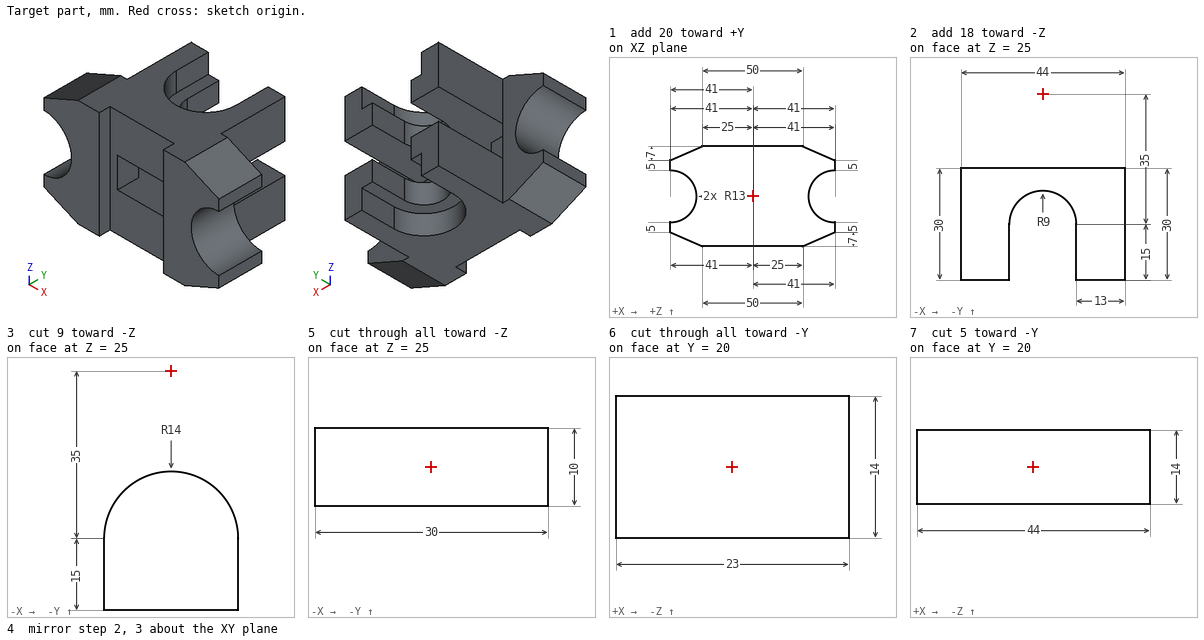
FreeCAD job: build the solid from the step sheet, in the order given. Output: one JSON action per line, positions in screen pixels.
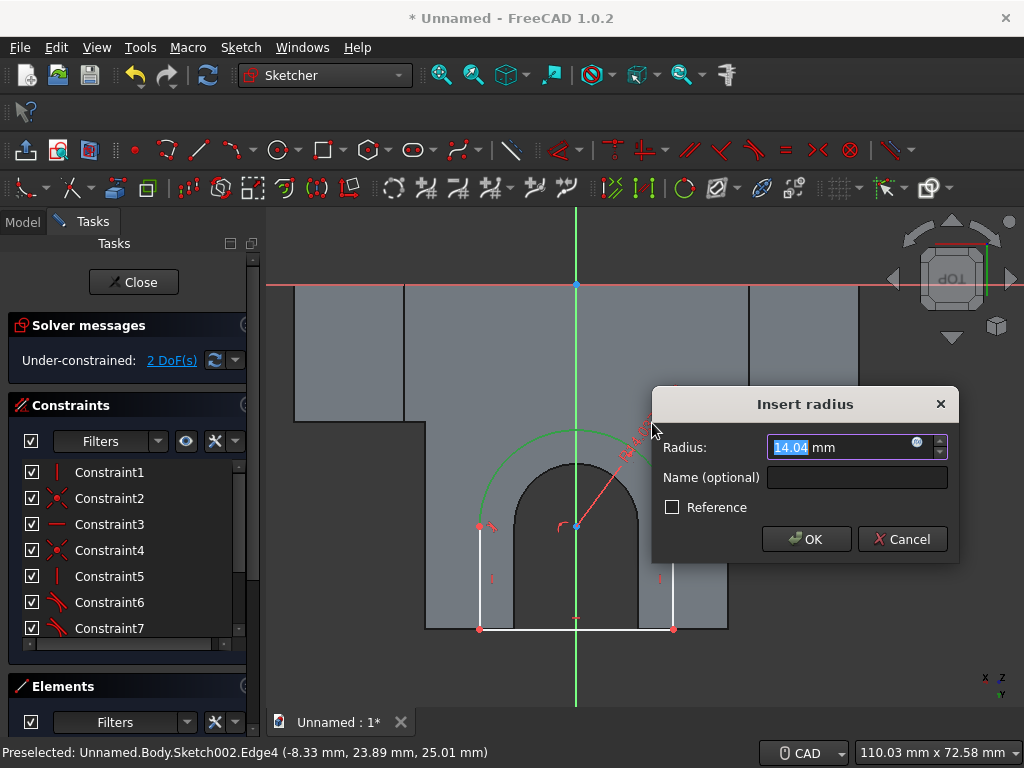
{"action": "type", "text": "14"}
{"action": "key", "text": "Return"}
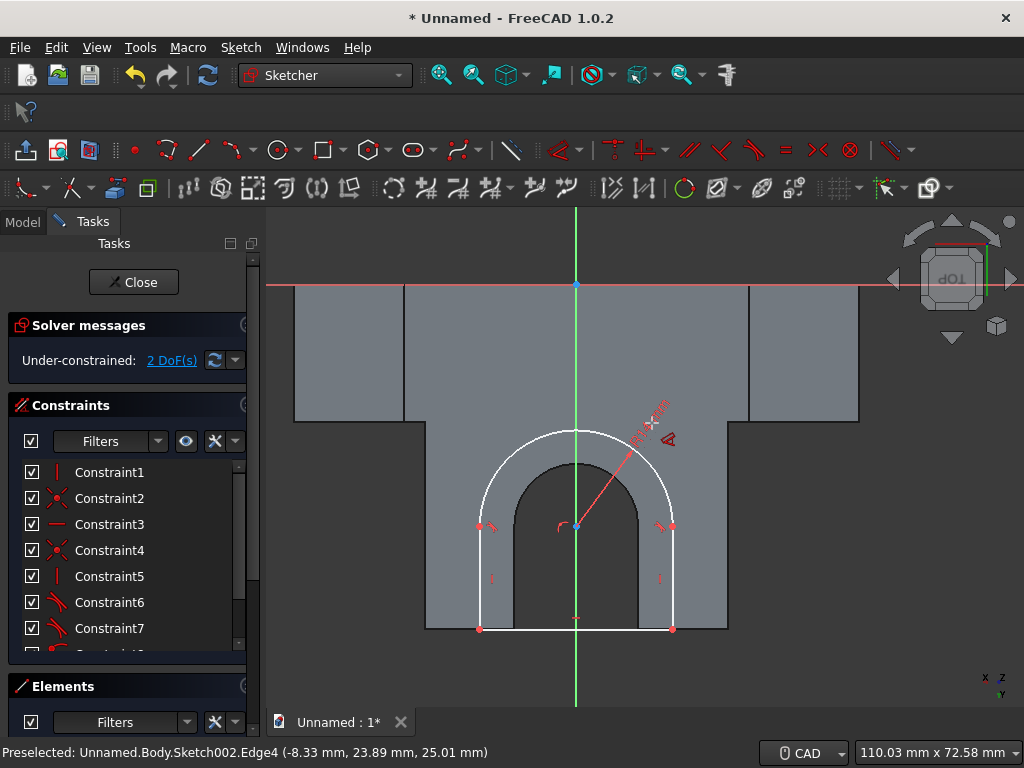
{"action": "left_click", "coordinate": [480, 558]}
{"action": "left_click", "coordinate": [446, 578]}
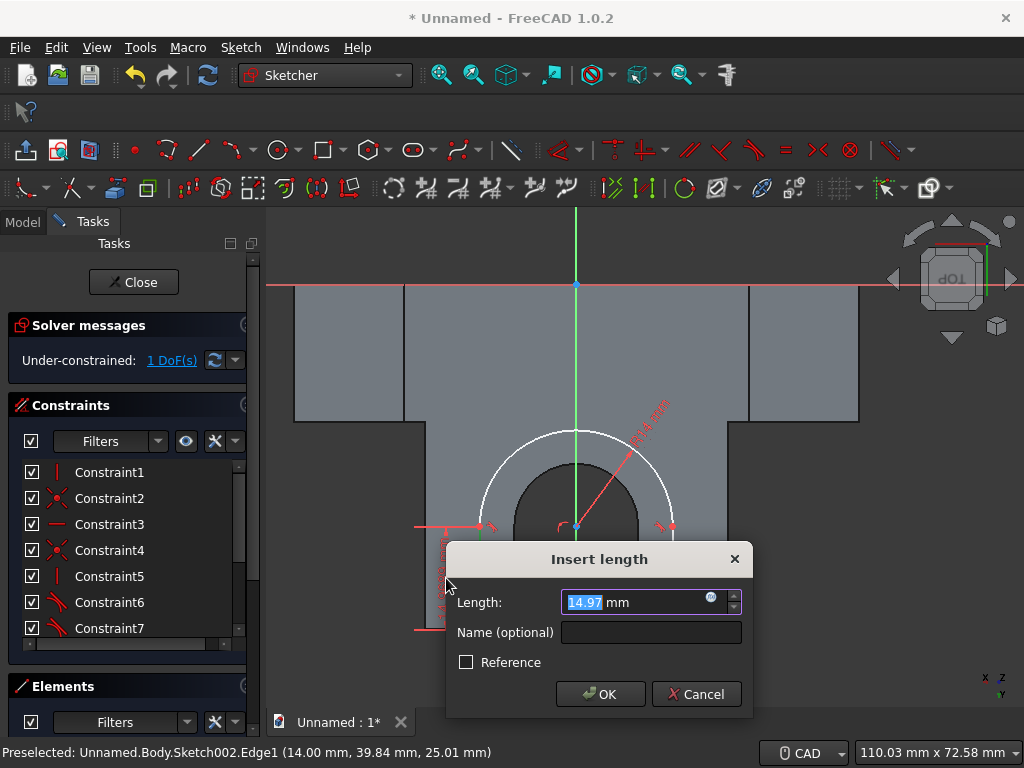
{"action": "type", "text": "15"}
{"action": "key", "text": "Return"}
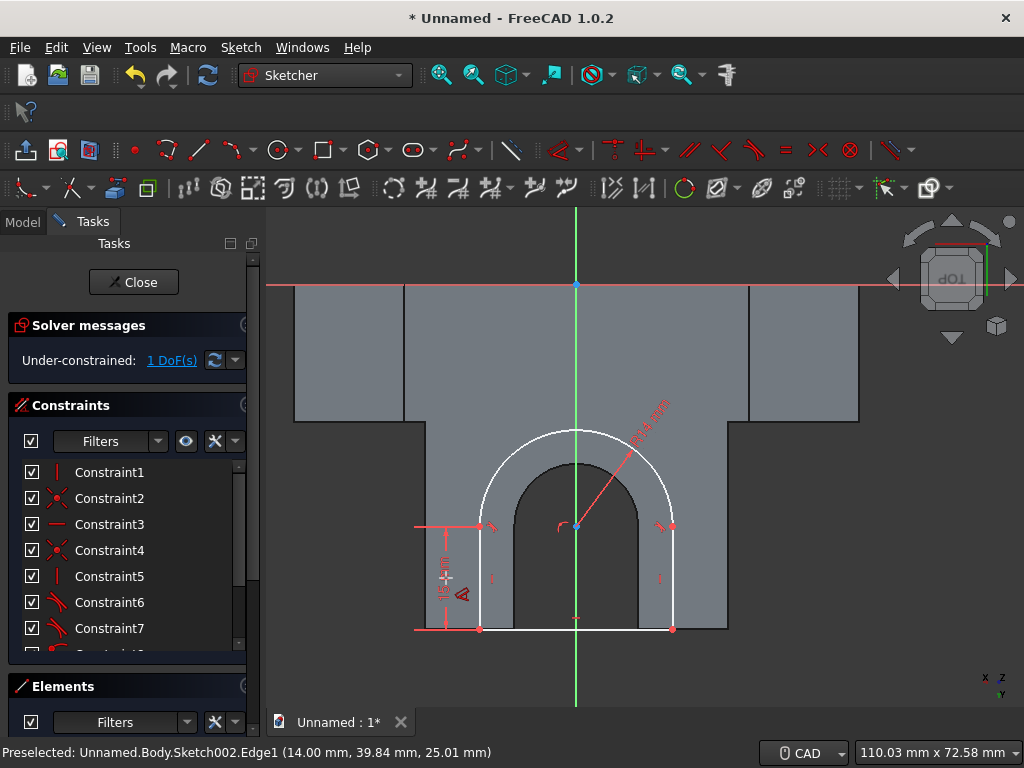
{"action": "left_click", "coordinate": [480, 527]}
{"action": "left_click", "coordinate": [446, 406]}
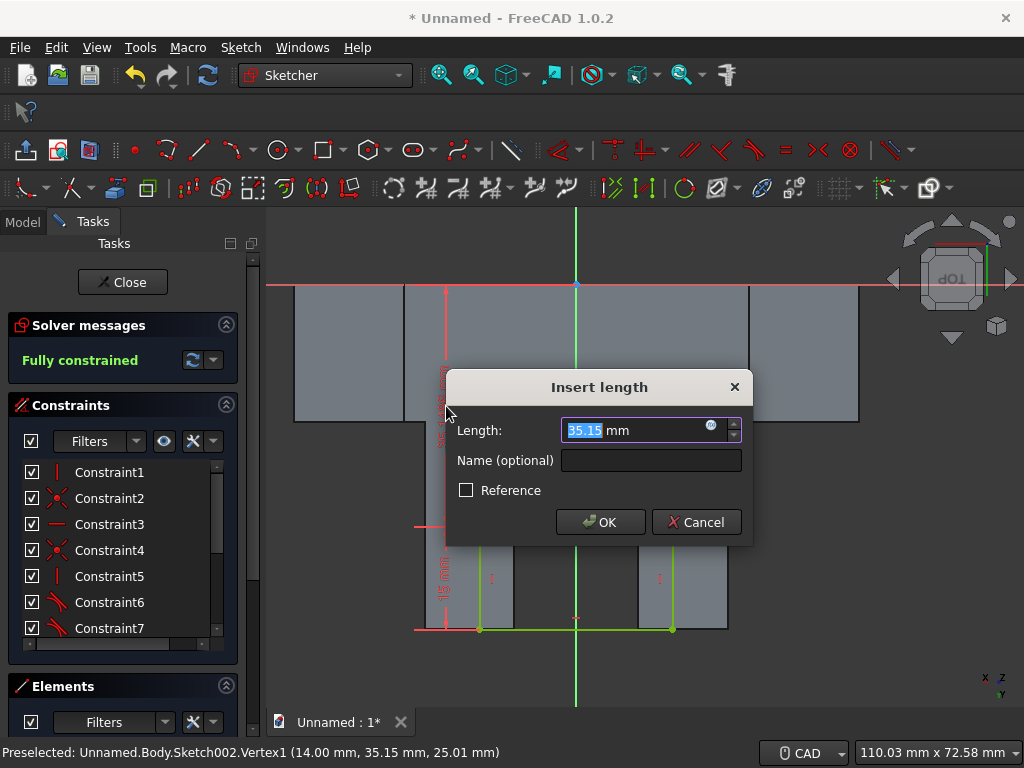
{"action": "type", "text": "35"}
{"action": "key", "text": "Return"}
{"action": "key", "text": "Escape"}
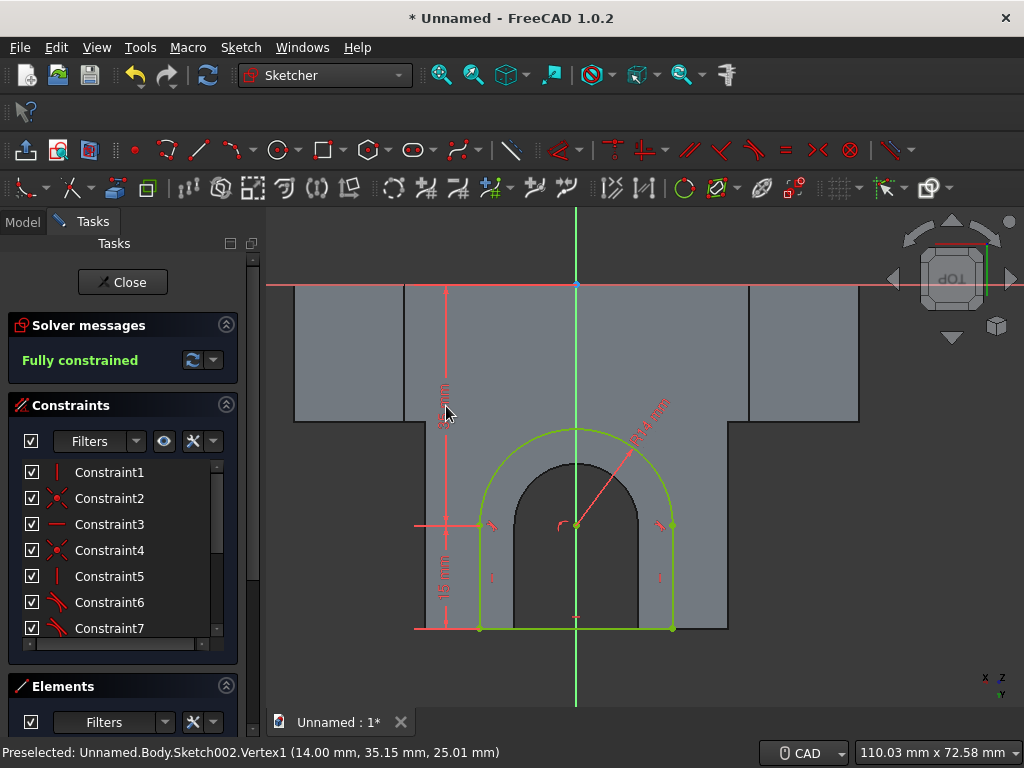
{"action": "left_click", "coordinate": [123, 282]}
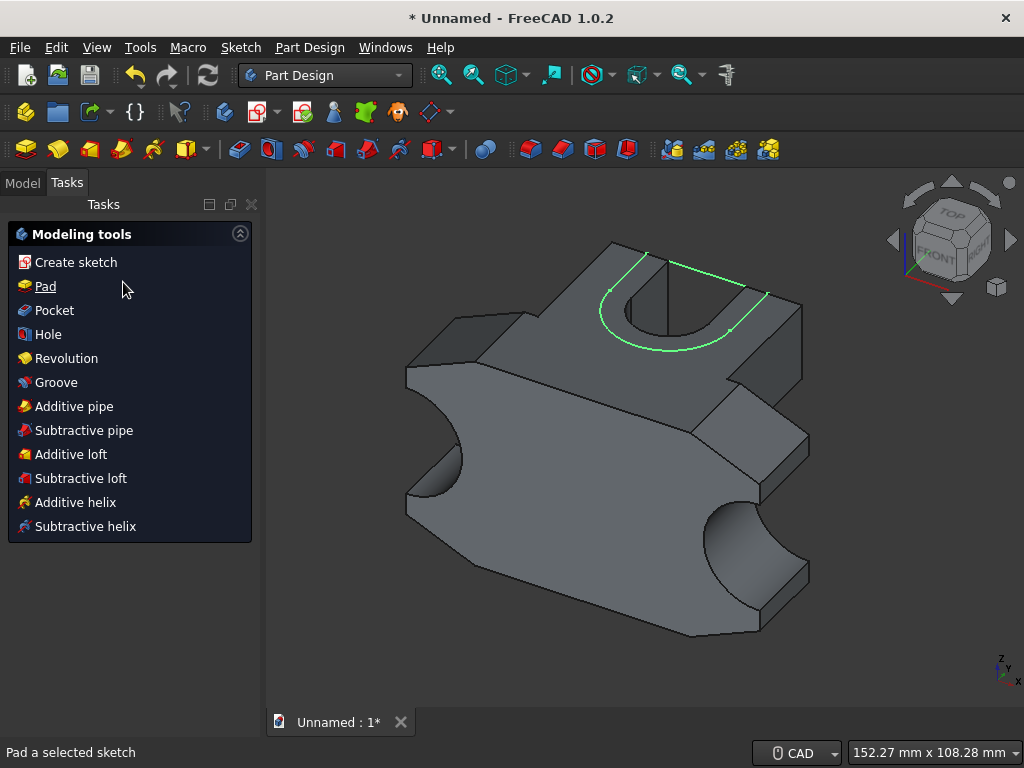
{"action": "left_click", "coordinate": [240, 150]}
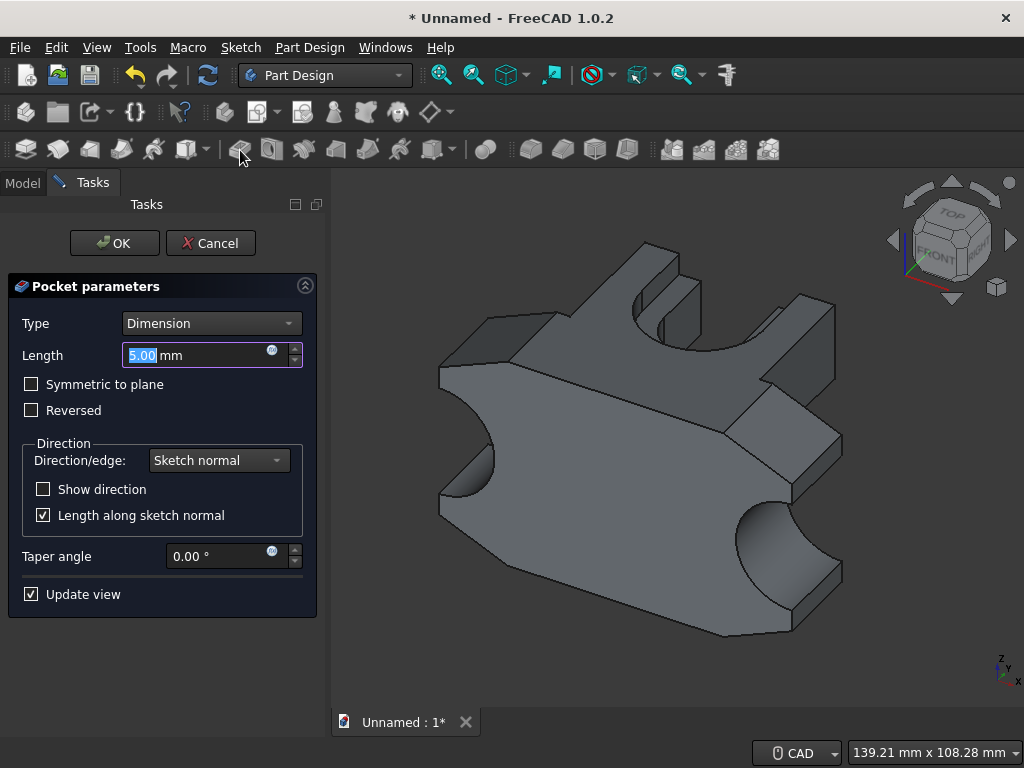
{"action": "type", "text": "9"}
{"action": "key", "text": "Tab"}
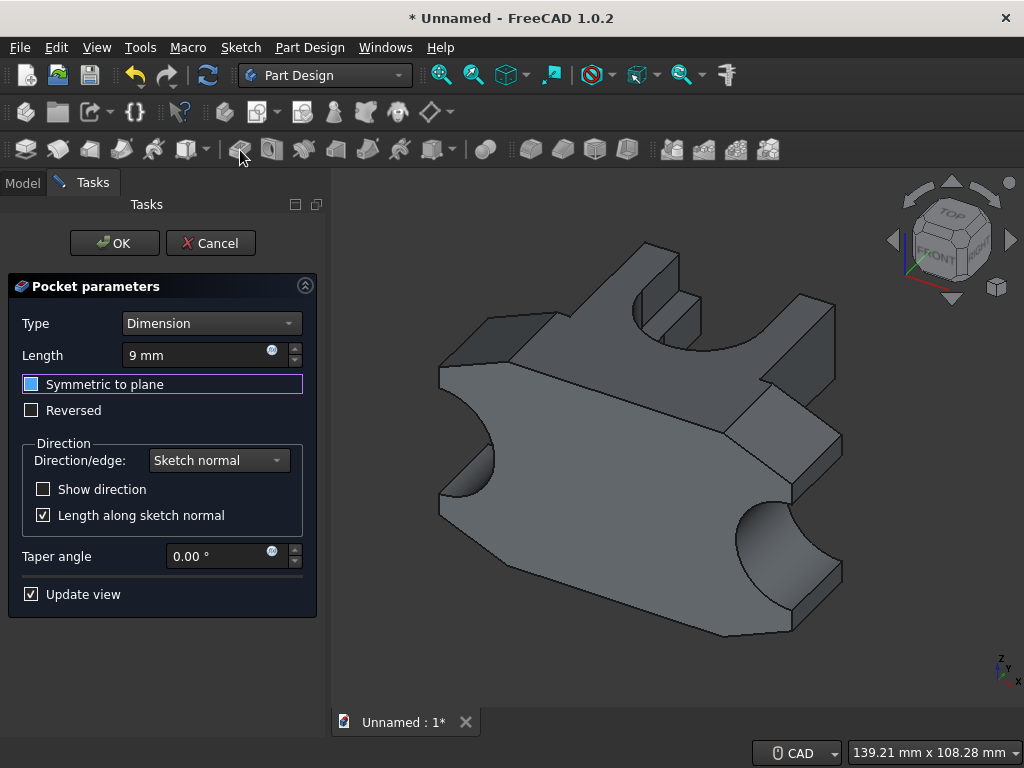
{"action": "left_click", "coordinate": [115, 243]}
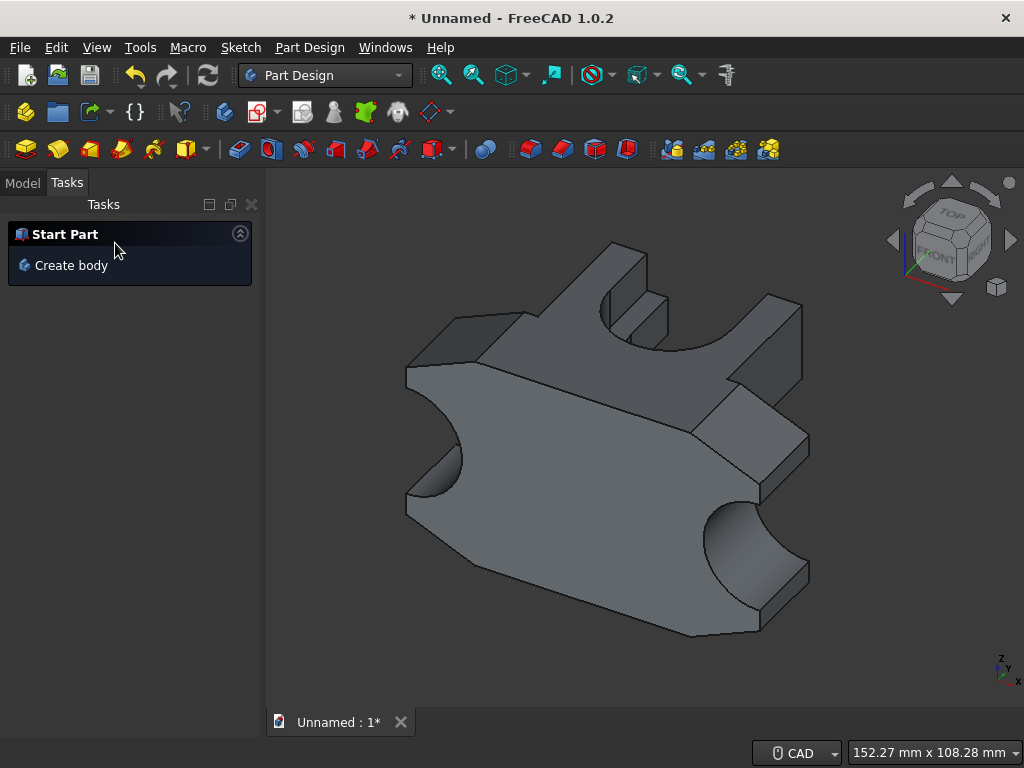
{"action": "left_click", "coordinate": [23, 182]}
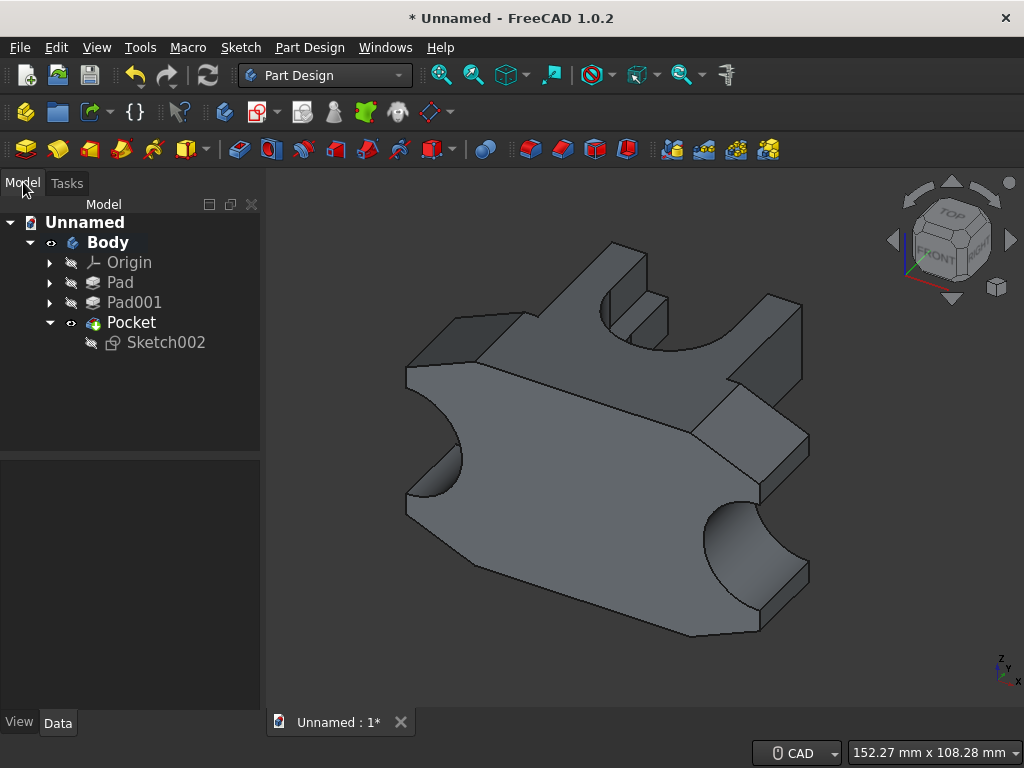
{"action": "left_click", "coordinate": [116, 303]}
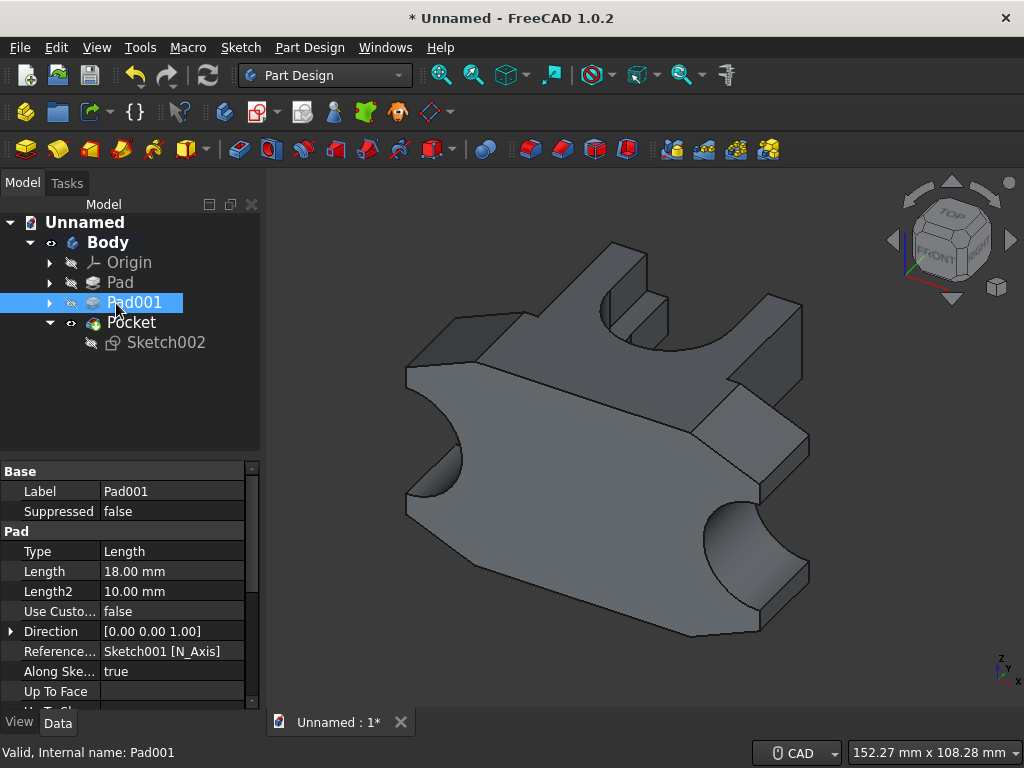
{"action": "left_click", "coordinate": [116, 323], "text": "ctrl"}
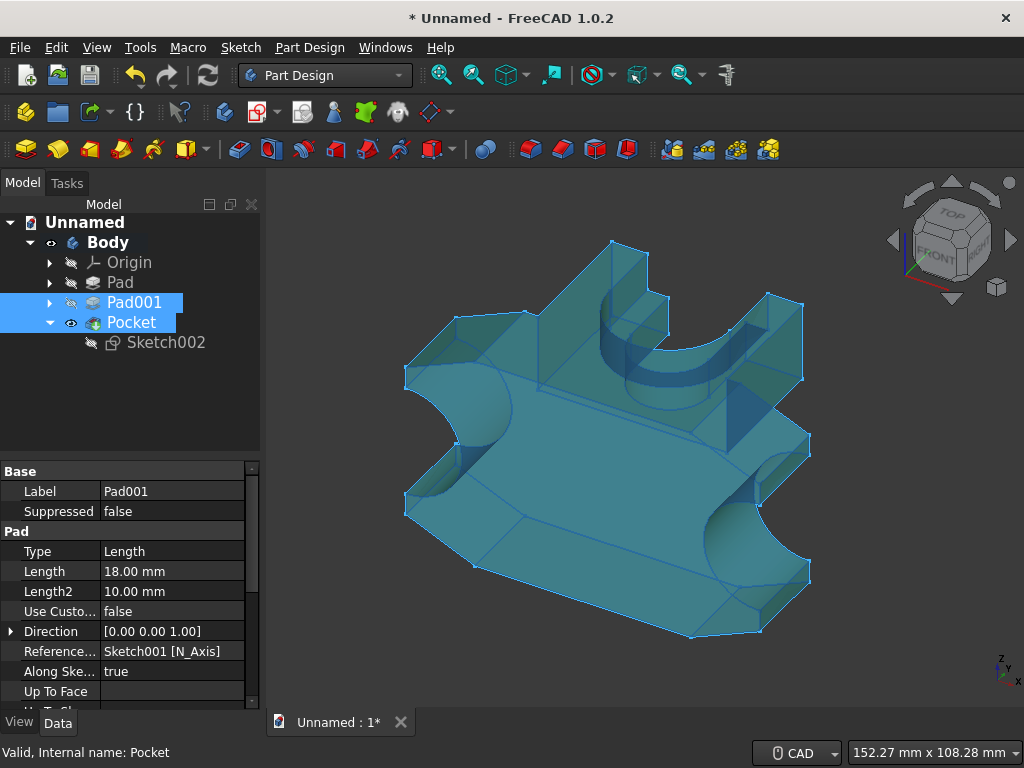
{"action": "left_click", "coordinate": [672, 150]}